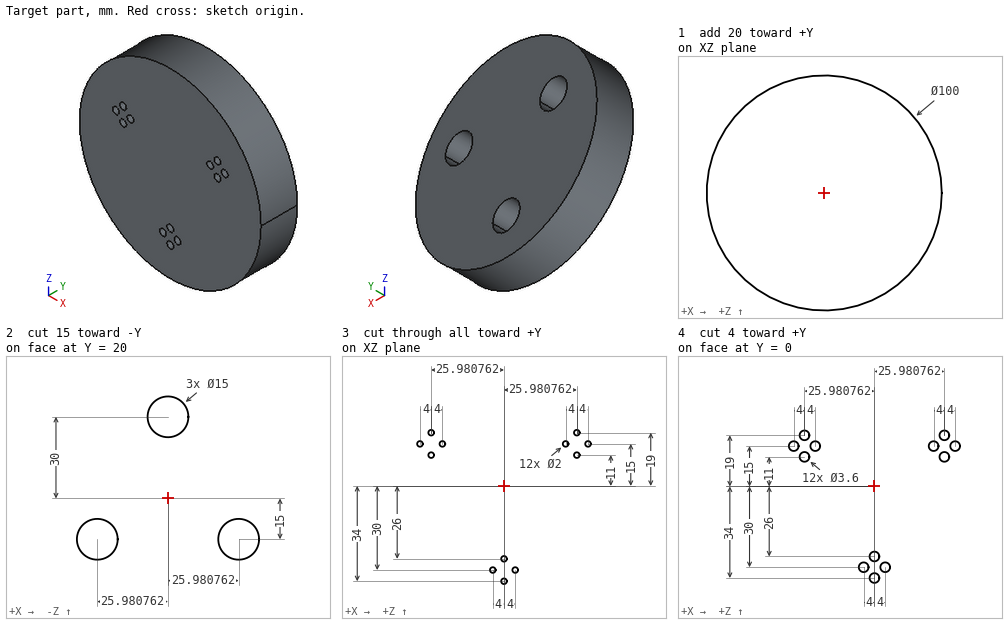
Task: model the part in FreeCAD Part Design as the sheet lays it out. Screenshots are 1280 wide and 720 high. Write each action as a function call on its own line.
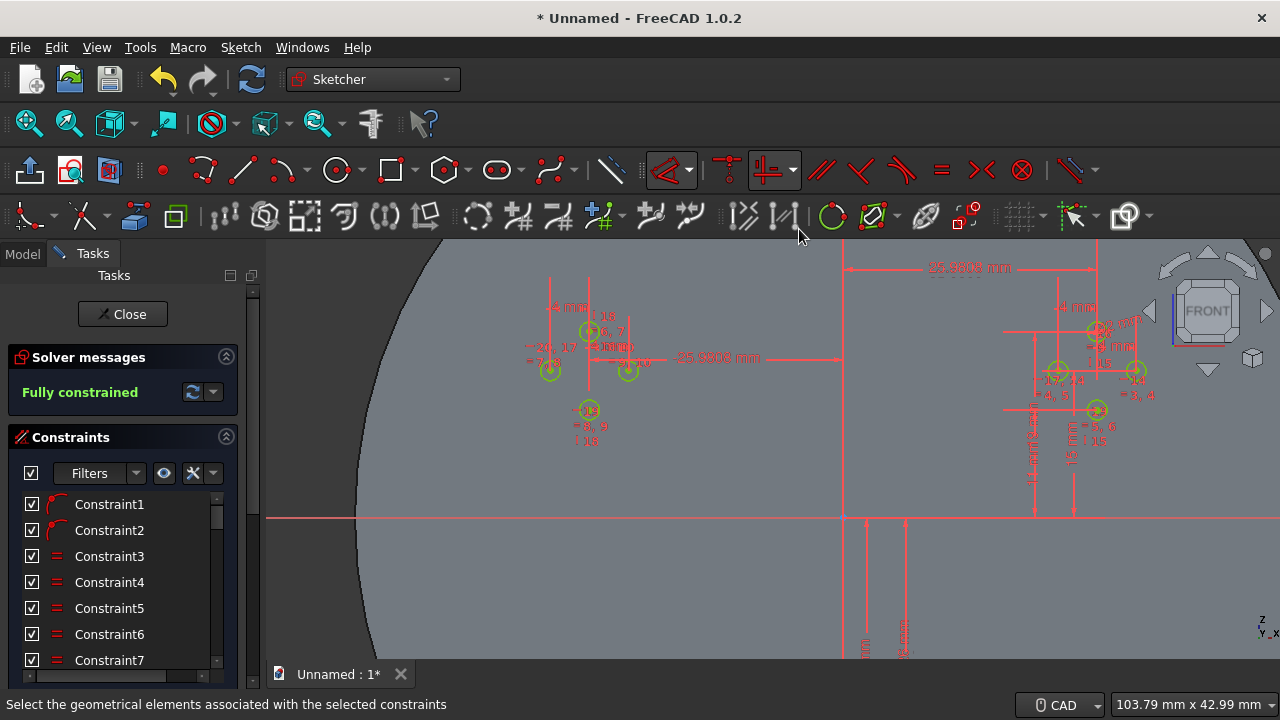
click(123, 314)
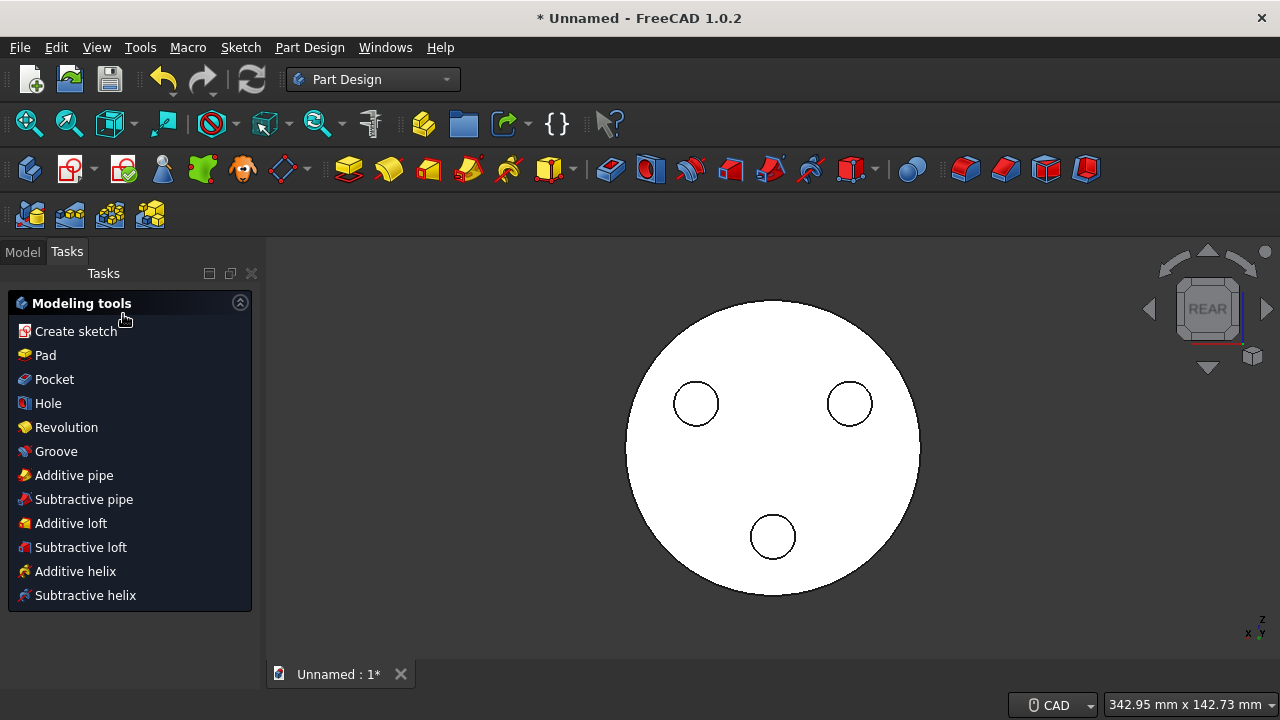
click(612, 170)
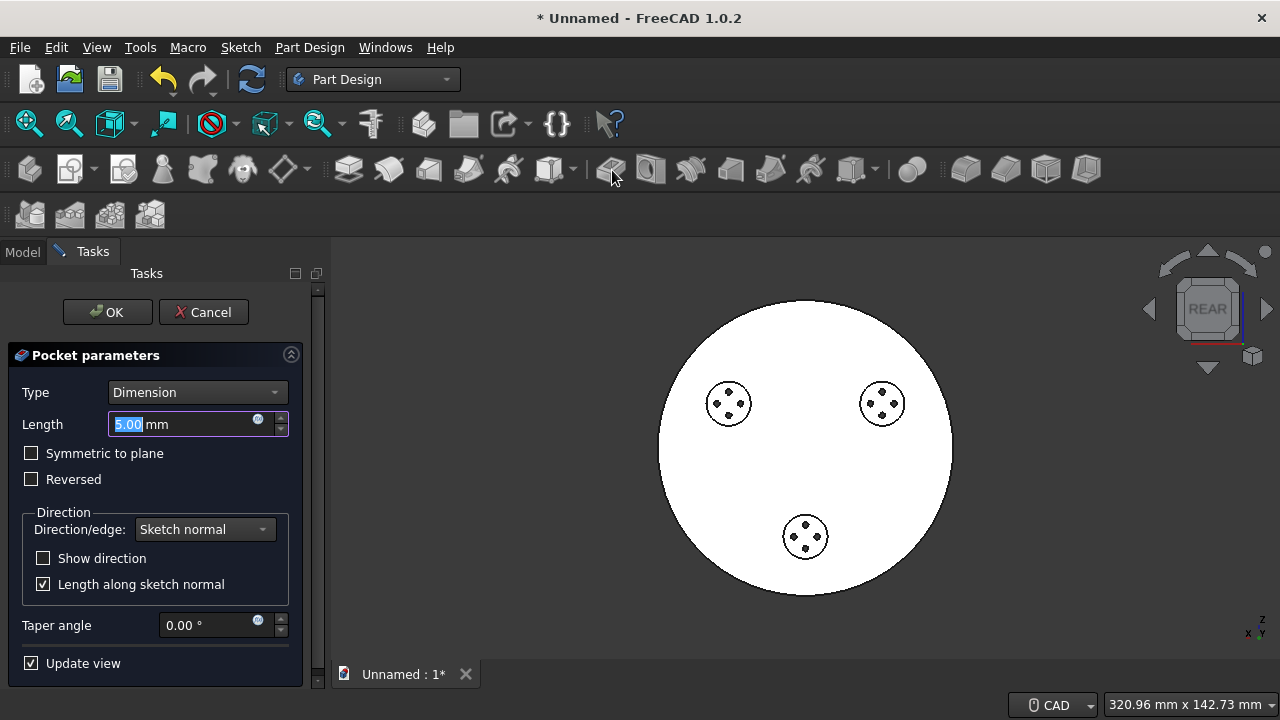
click(198, 392)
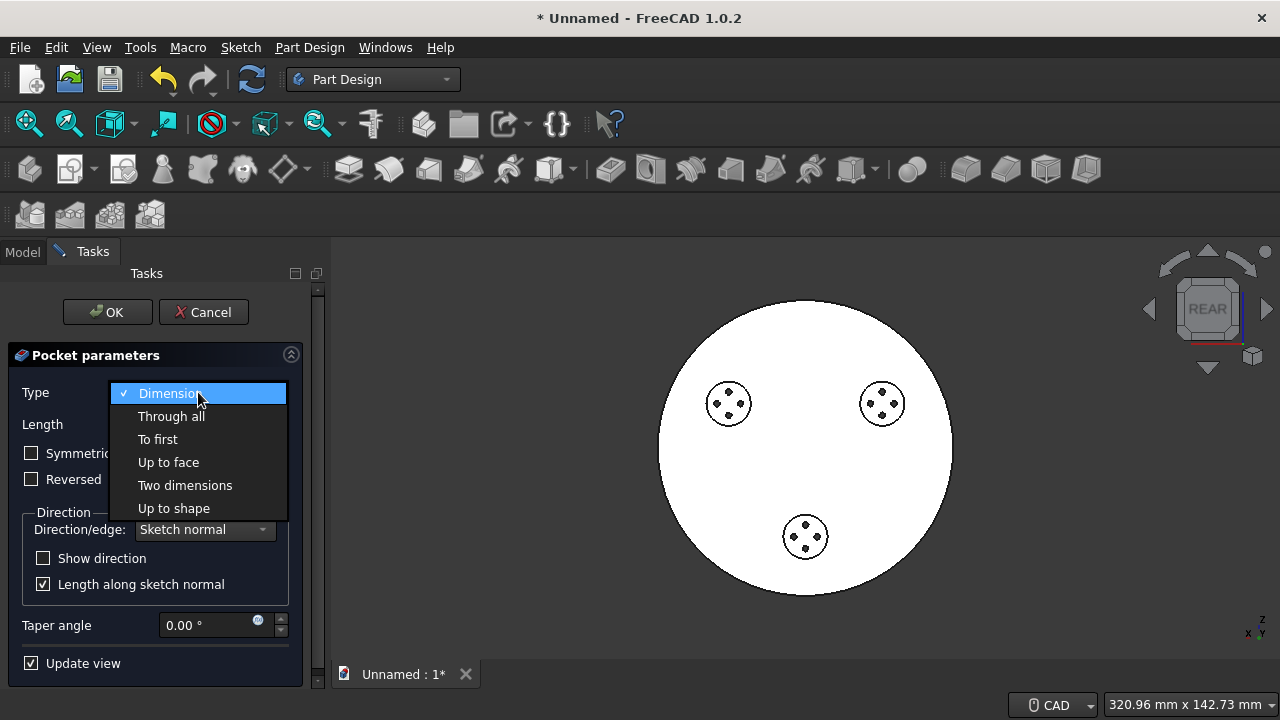
click(198, 416)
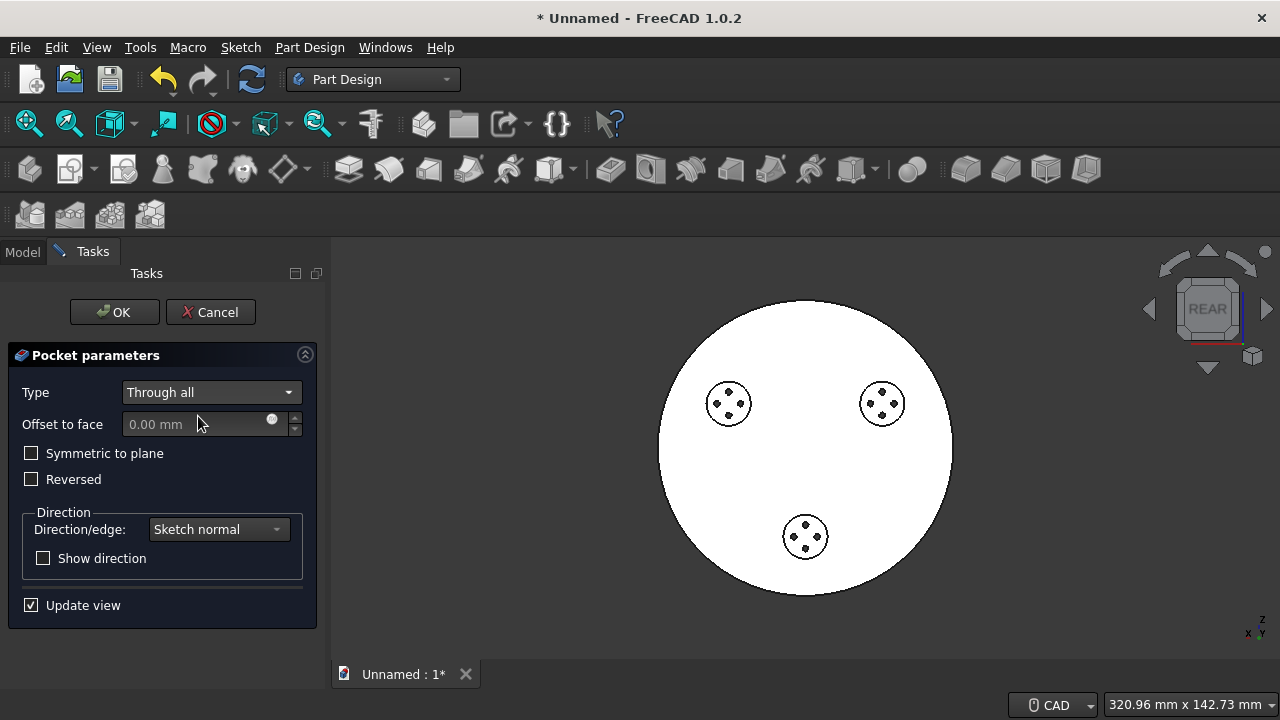
click(115, 312)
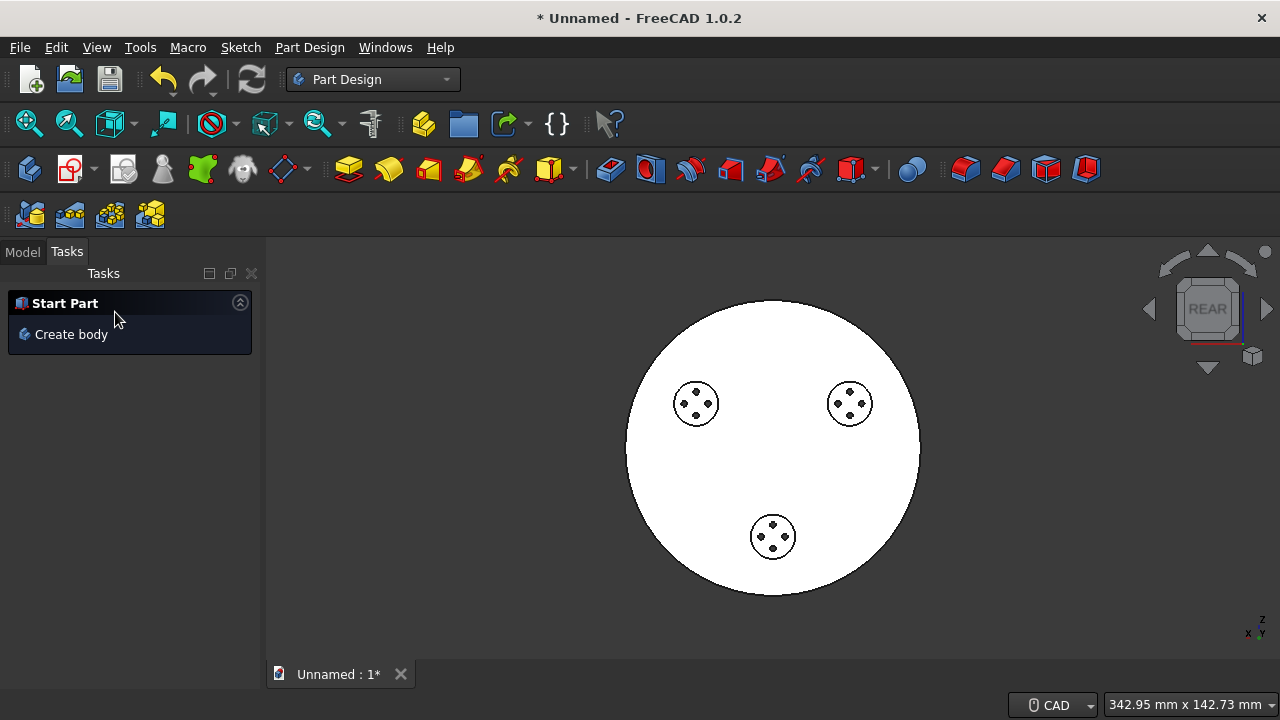
key(0)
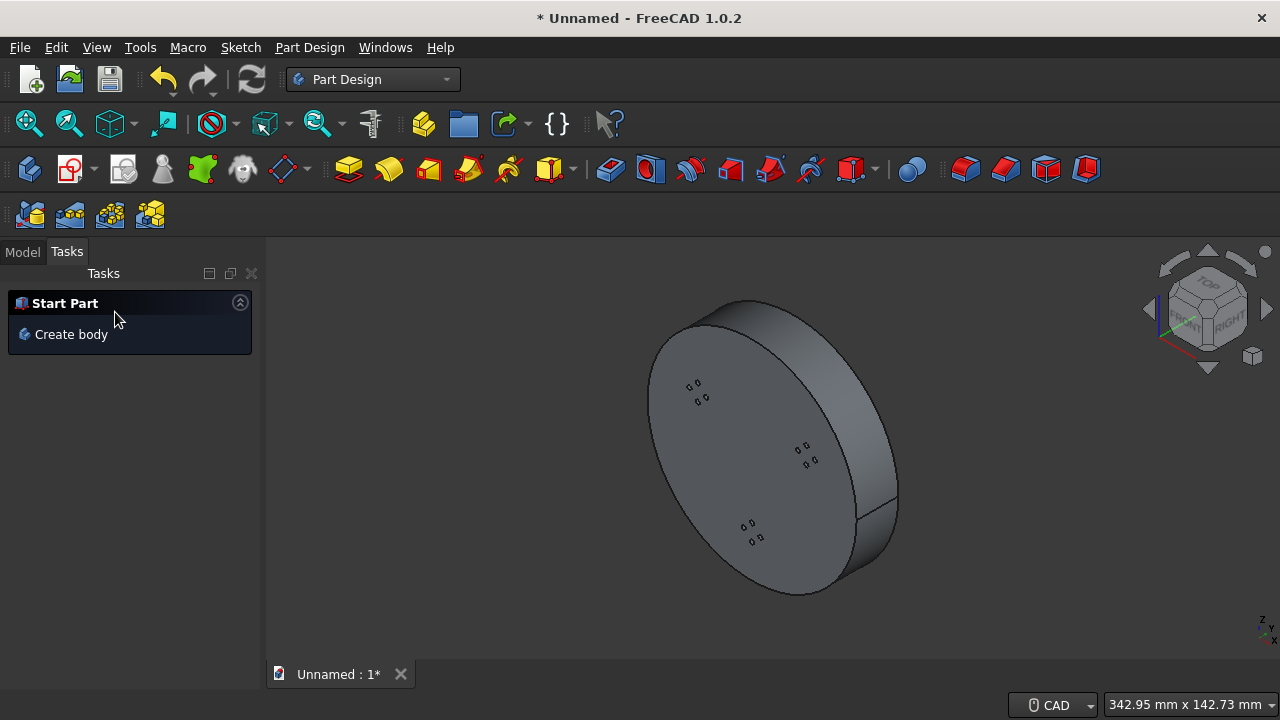
click(752, 459)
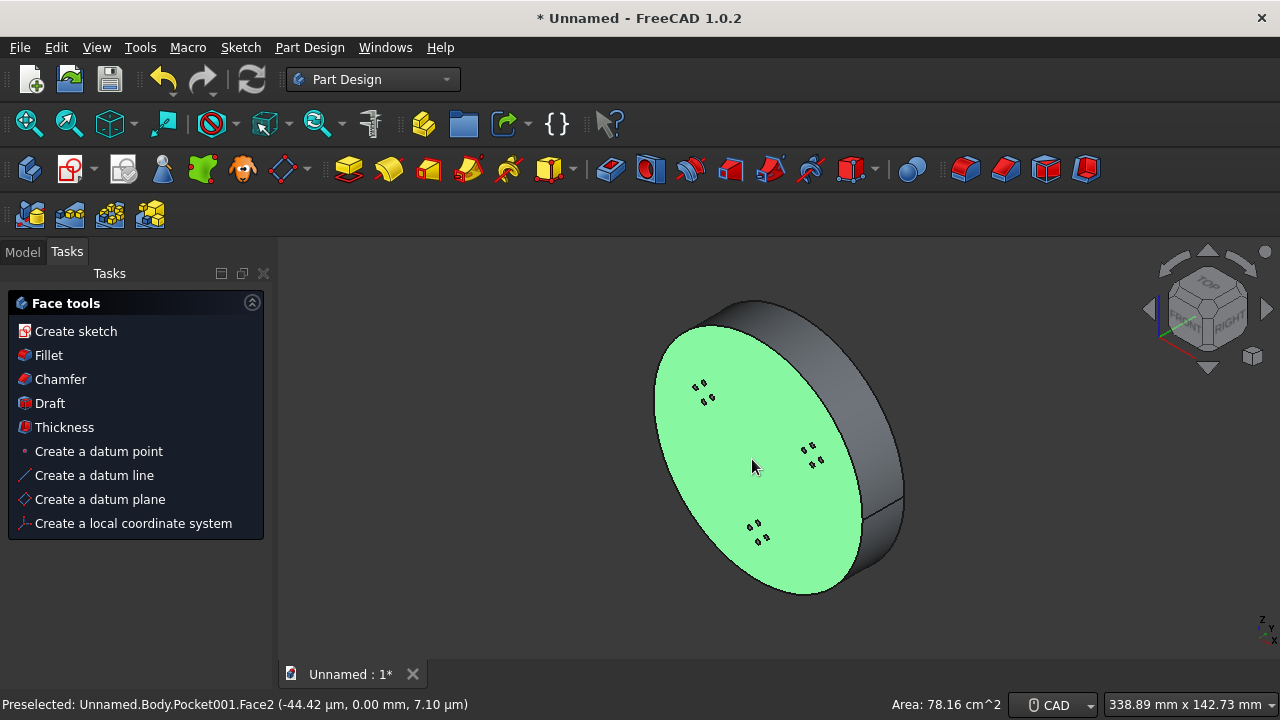
click(70, 170)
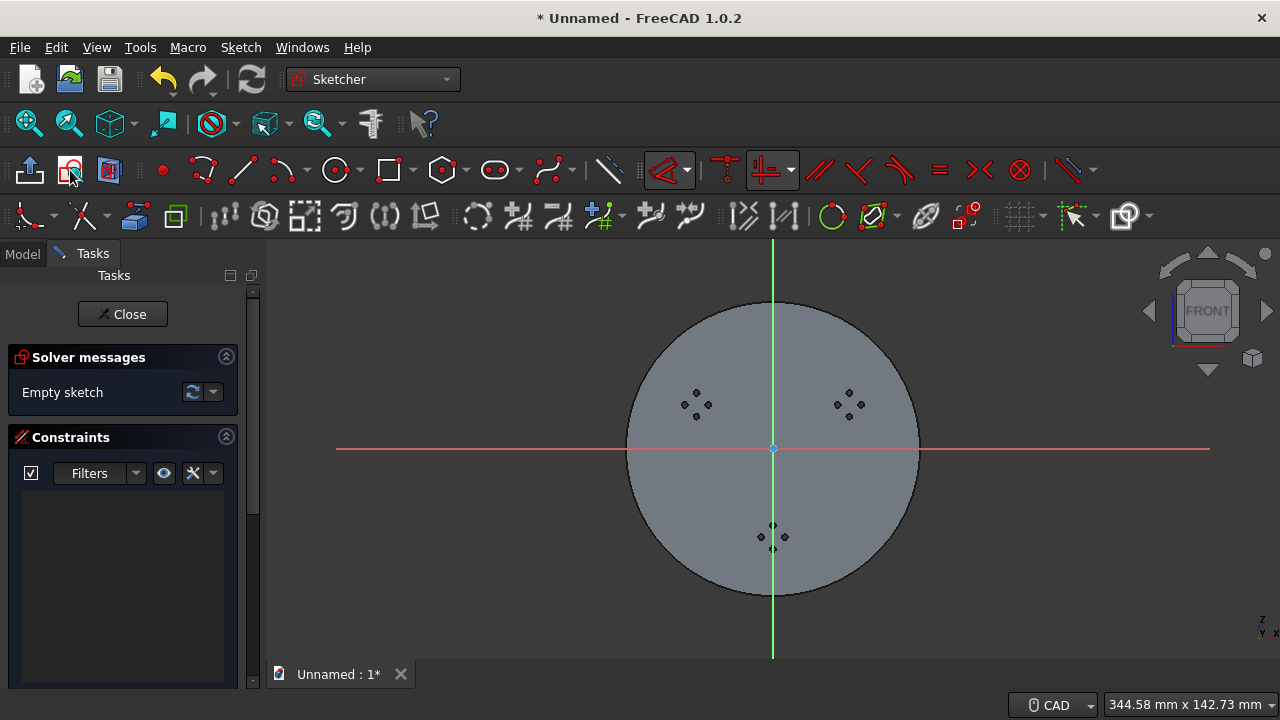
scroll(912, 516, up, 2)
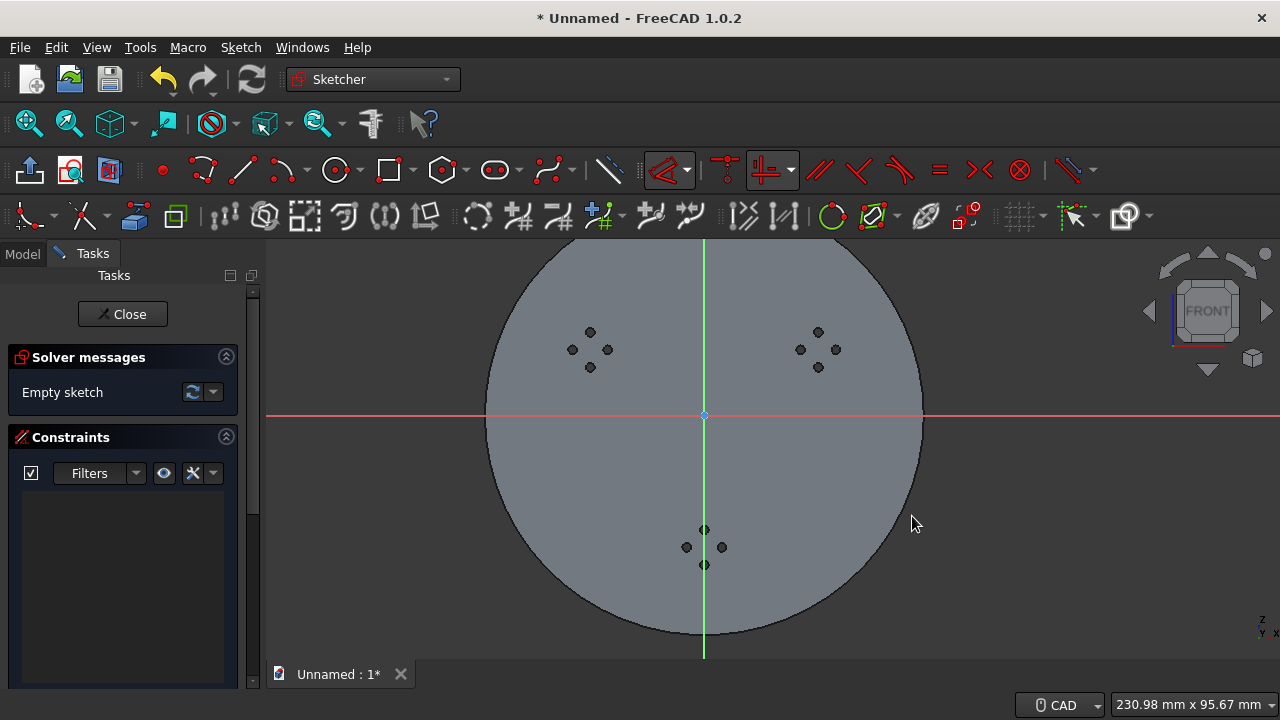
click(336, 170)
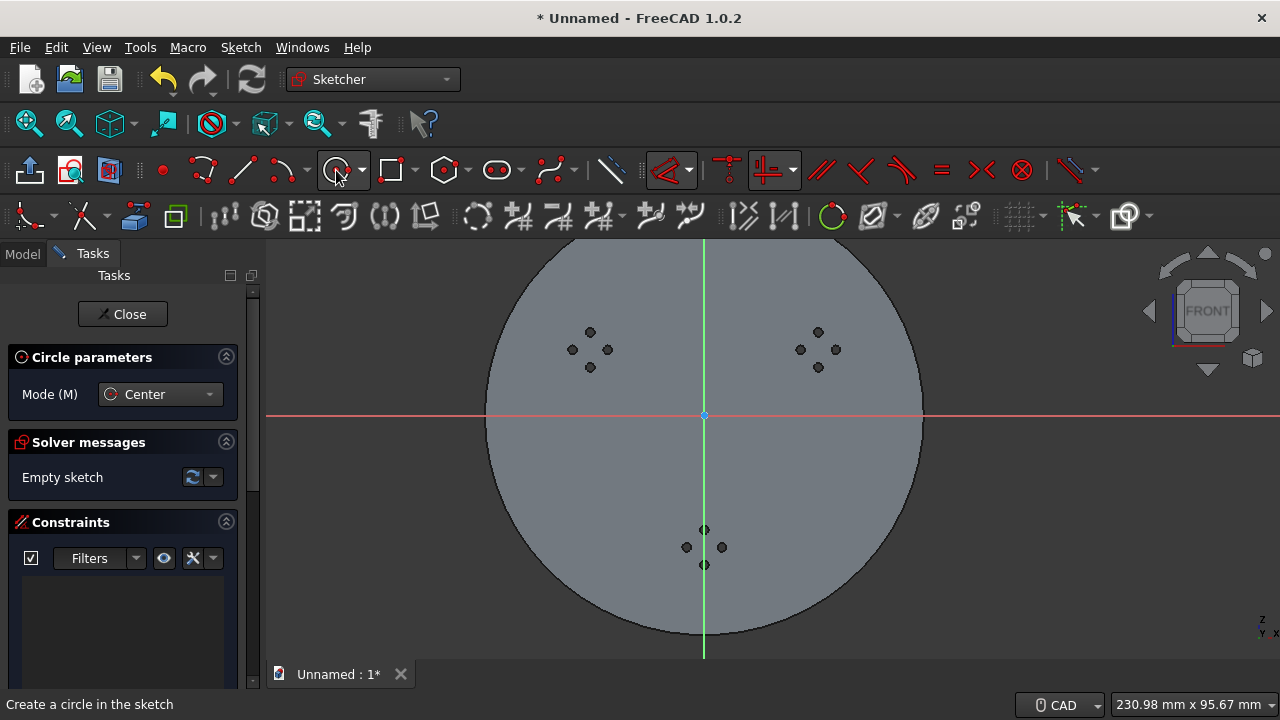
scroll(590, 332, up, 6)